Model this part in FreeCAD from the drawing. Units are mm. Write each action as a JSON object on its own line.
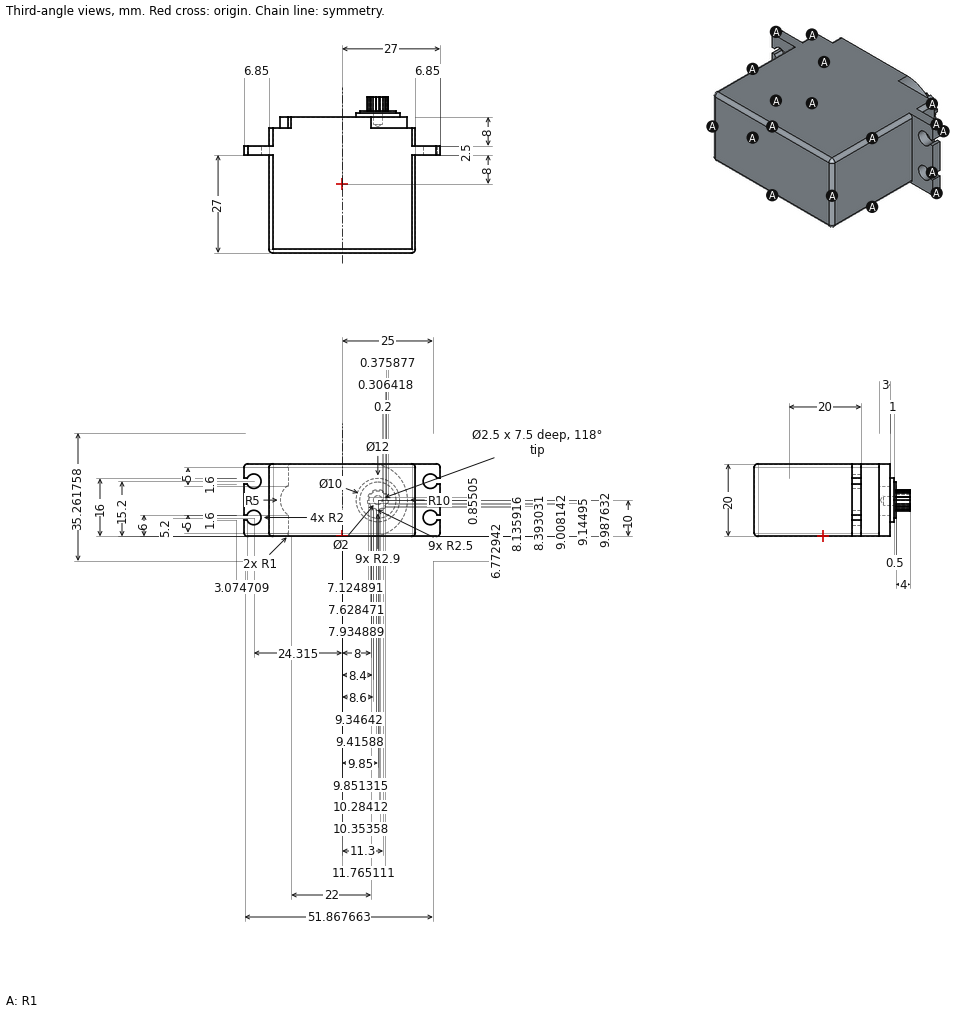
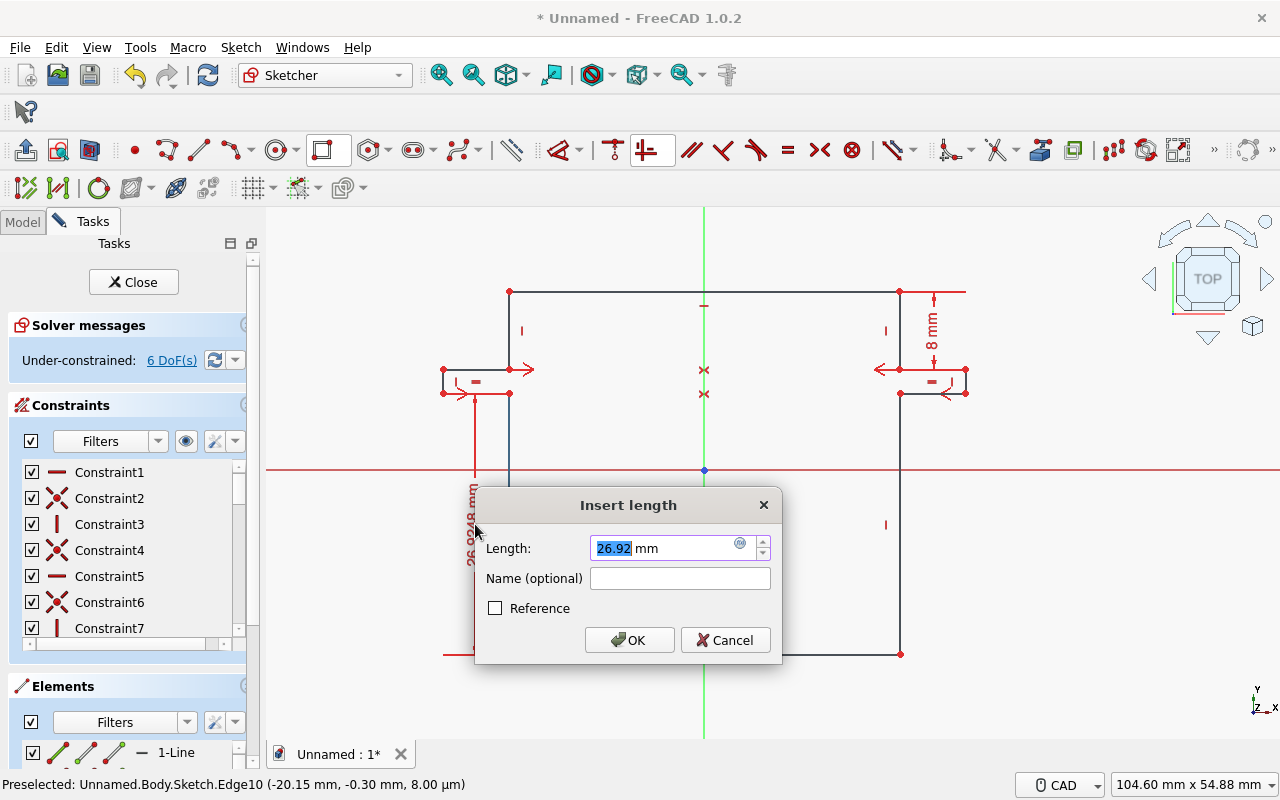
{"action": "type", "text": "27"}
{"action": "key", "text": "Return"}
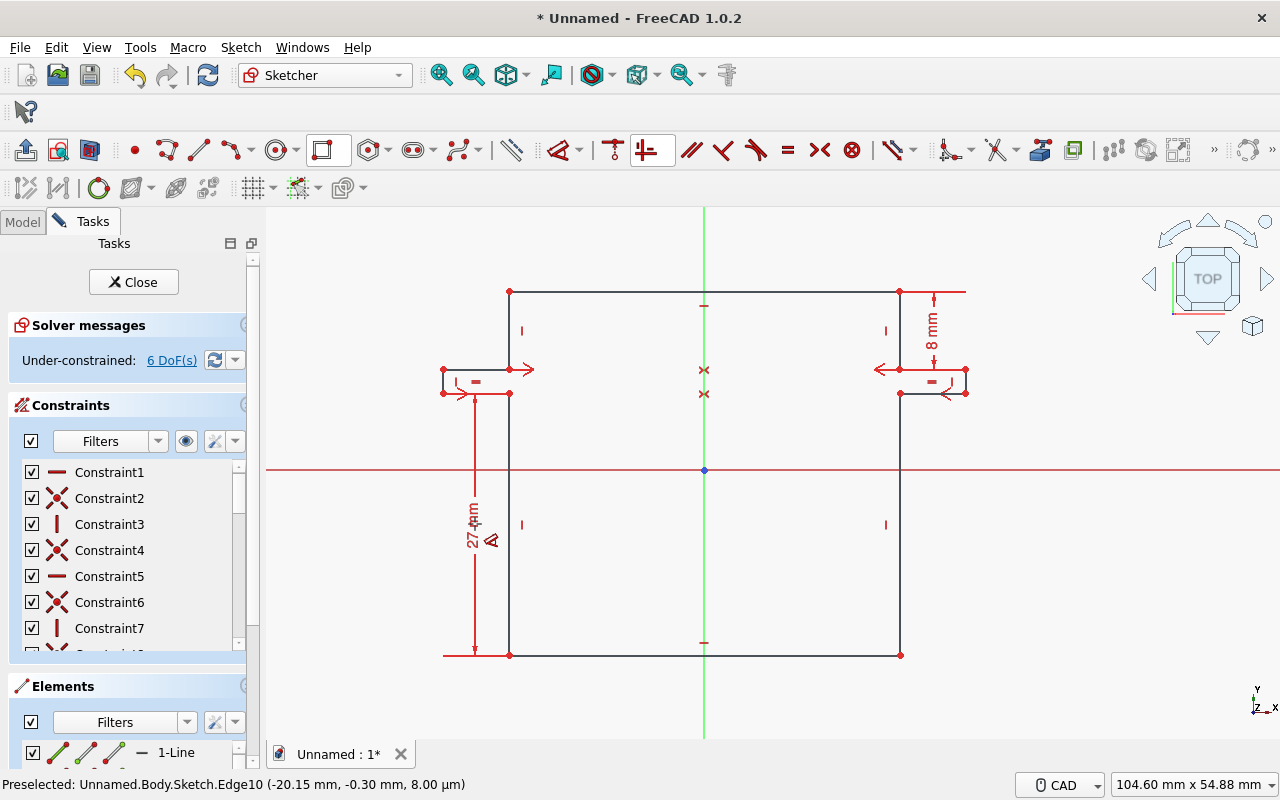
{"action": "left_click", "coordinate": [900, 394]}
{"action": "left_click", "coordinate": [934, 432]}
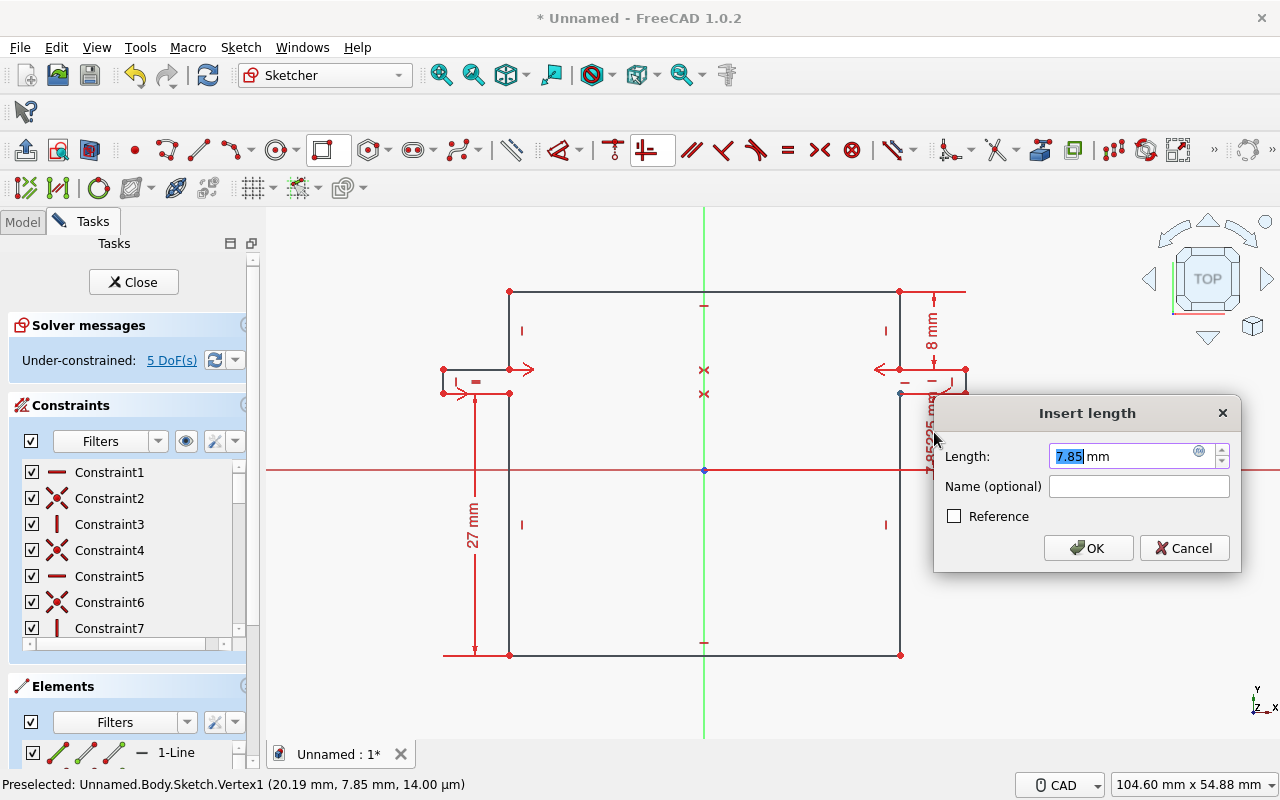
{"action": "type", "text": "8"}
{"action": "key", "text": "Return"}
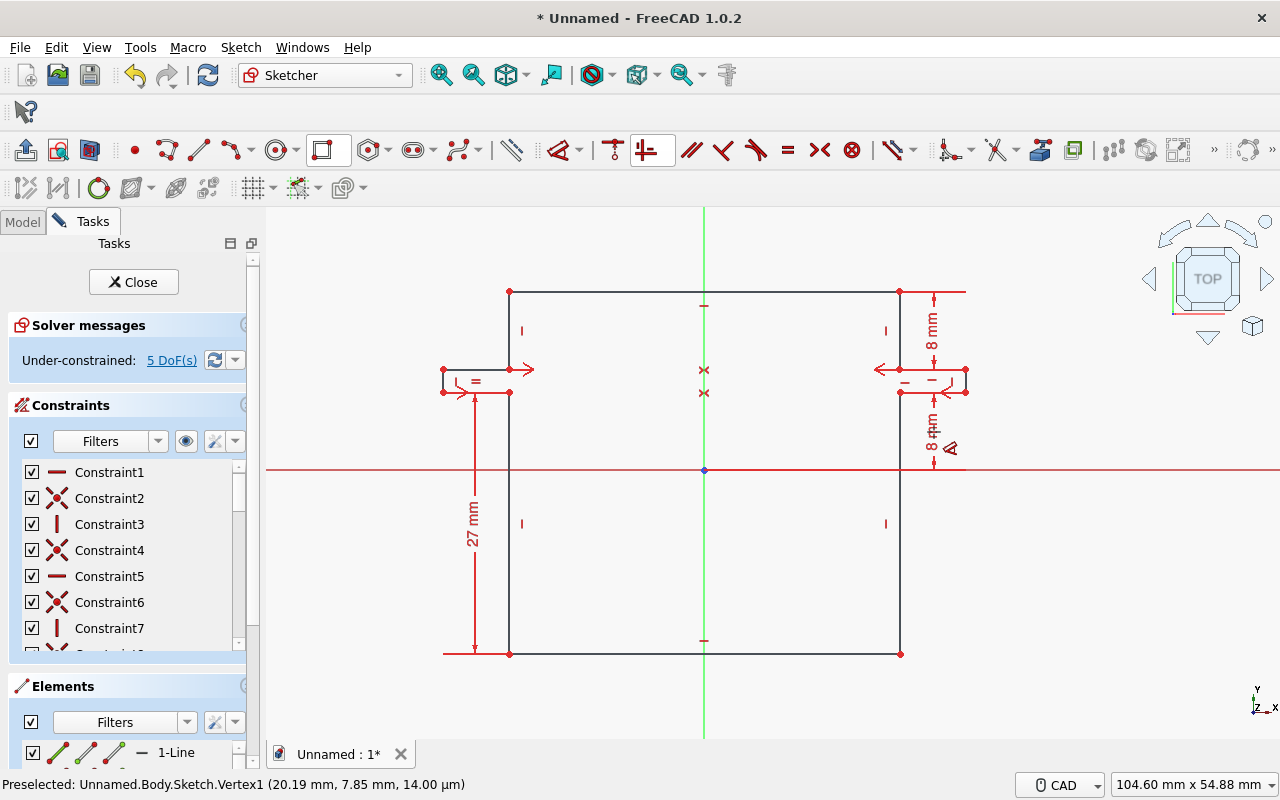
{"action": "scroll", "coordinate": [966, 383], "scroll_direction": "up", "scroll_amount": 3}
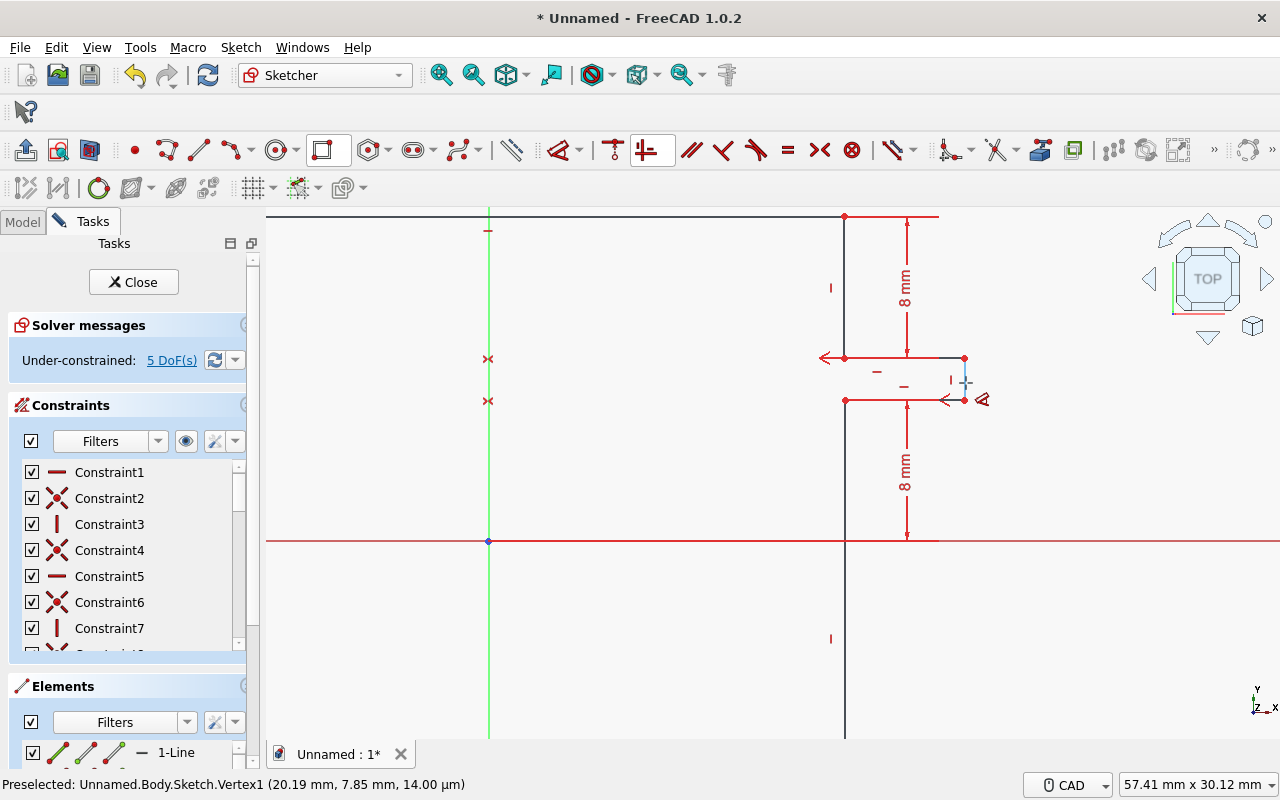
{"action": "left_click", "coordinate": [965, 383]}
{"action": "left_click", "coordinate": [999, 379]}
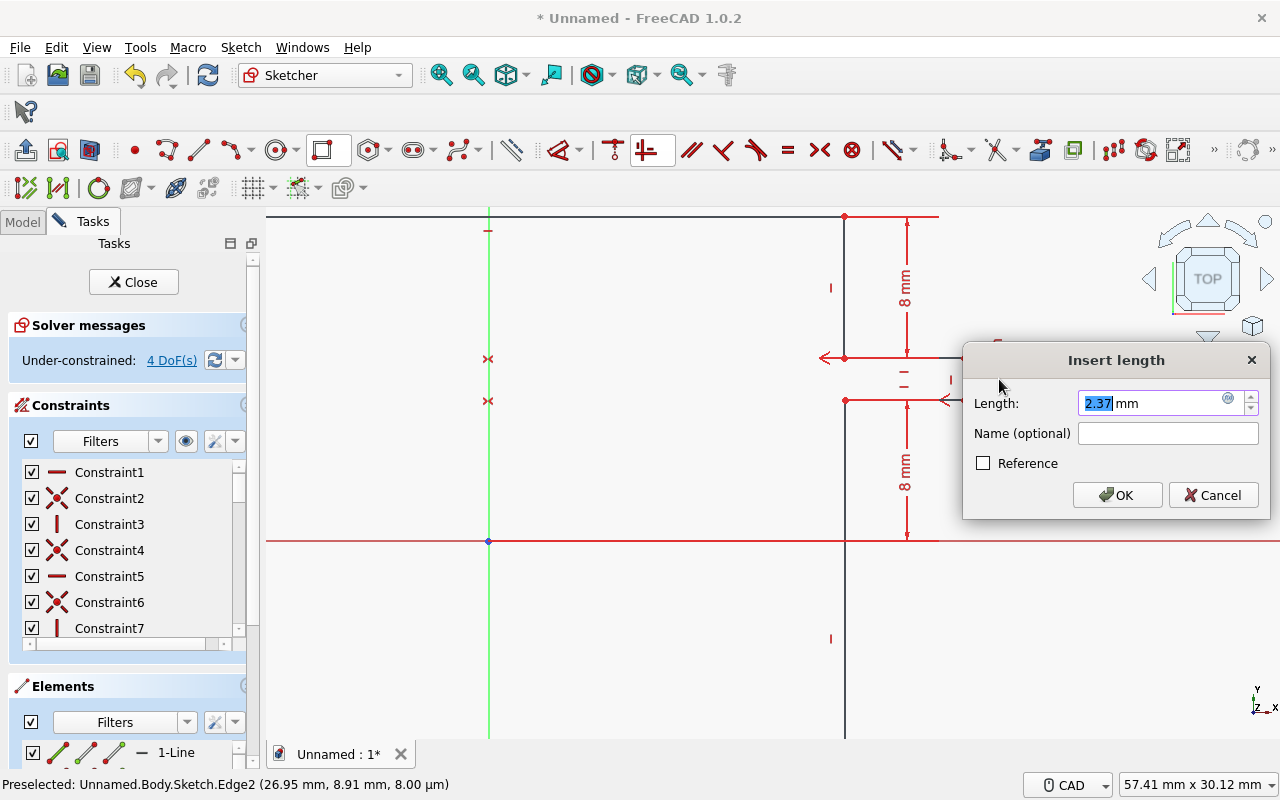
{"action": "type", "text": "2.5"}
{"action": "key", "text": "Return"}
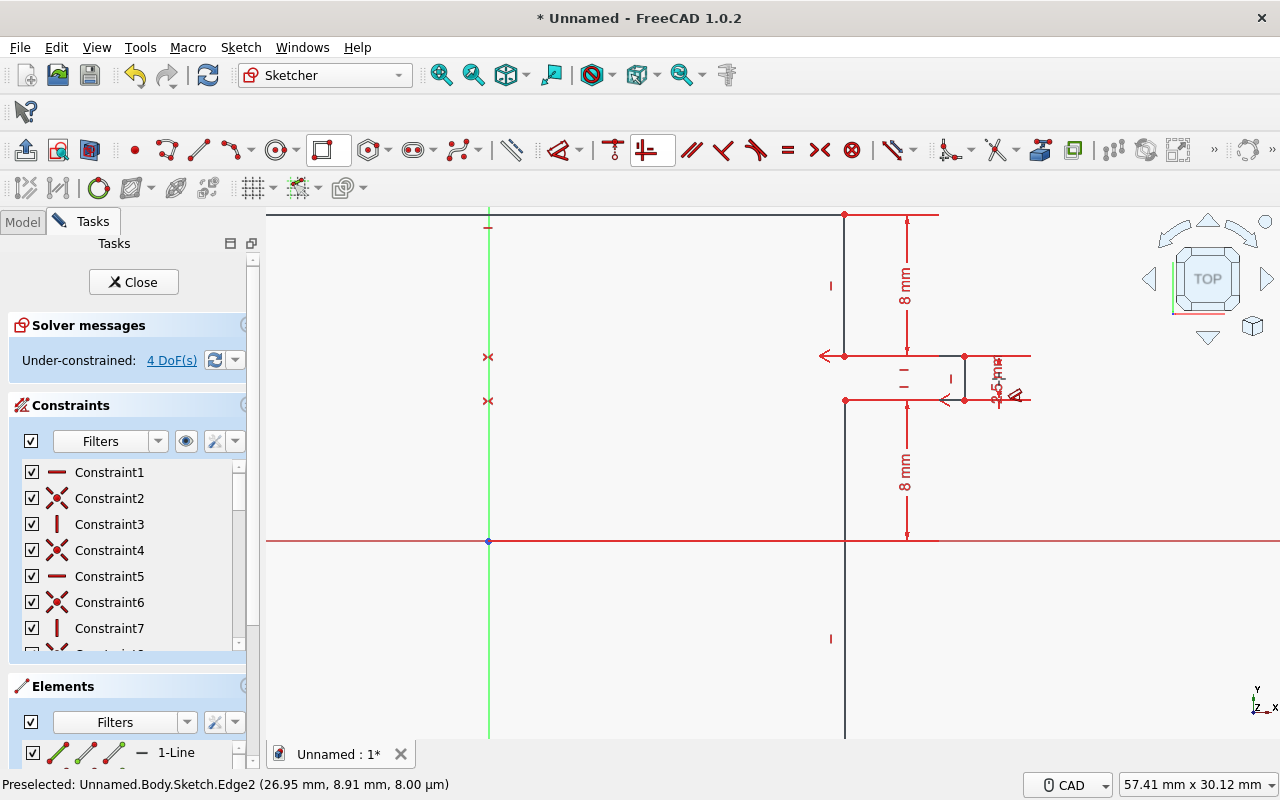
{"action": "left_click", "coordinate": [965, 400]}
{"action": "left_click", "coordinate": [727, 366]}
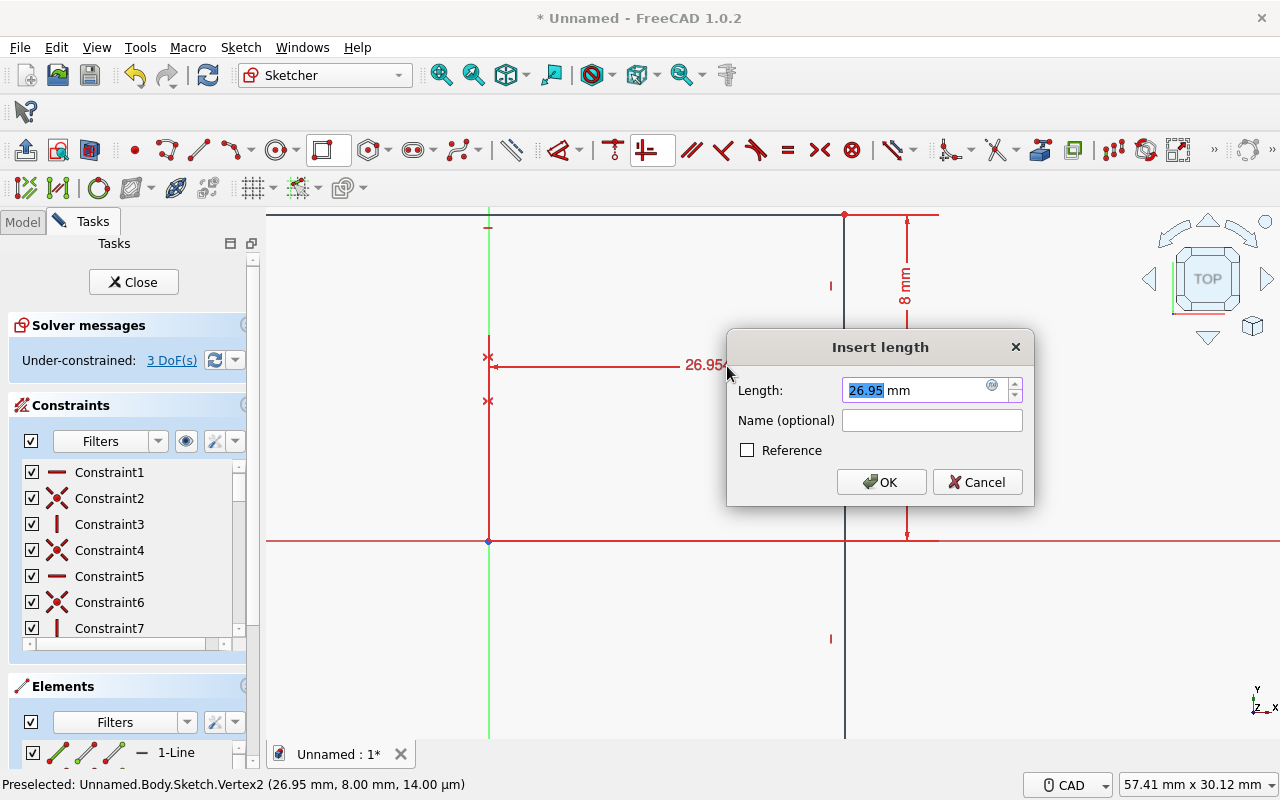
{"action": "type", "text": "27"}
{"action": "key", "text": "Return"}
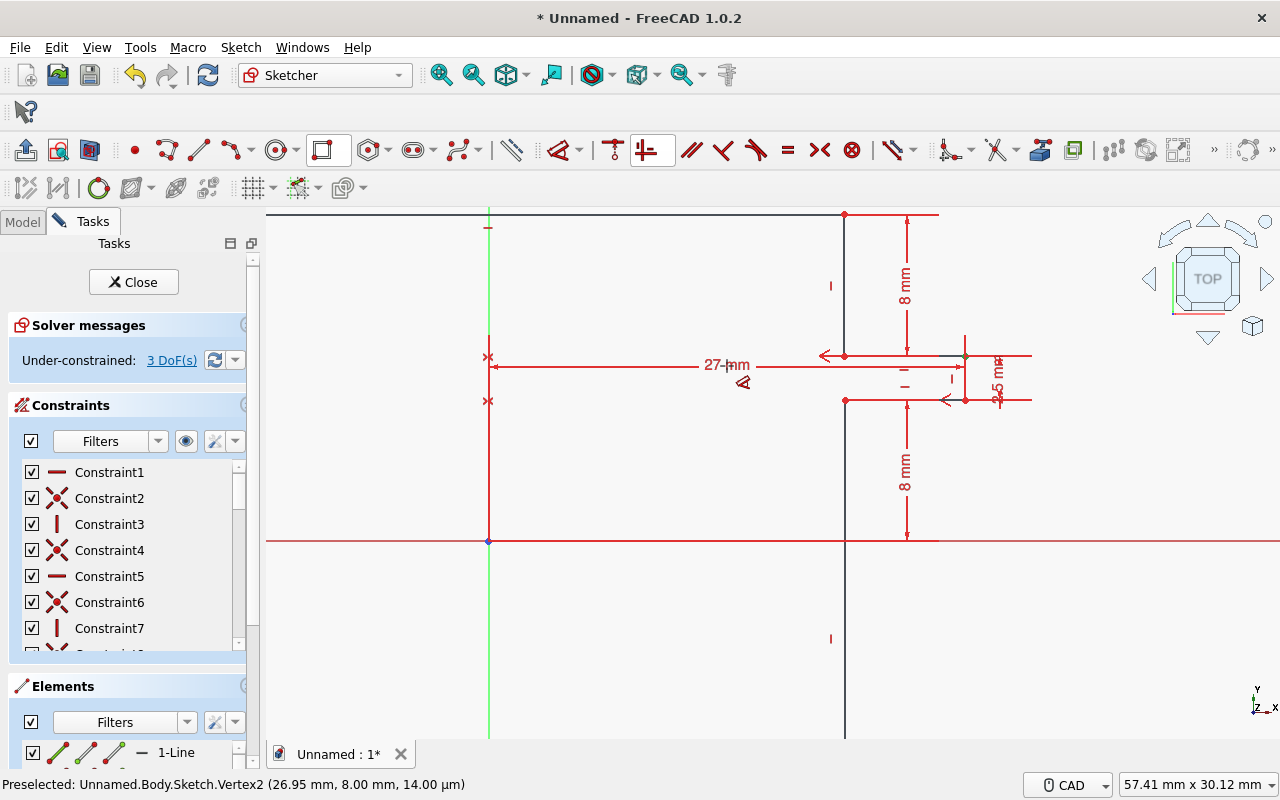
{"action": "left_click", "coordinate": [881, 400]}
{"action": "left_click", "coordinate": [905, 434]}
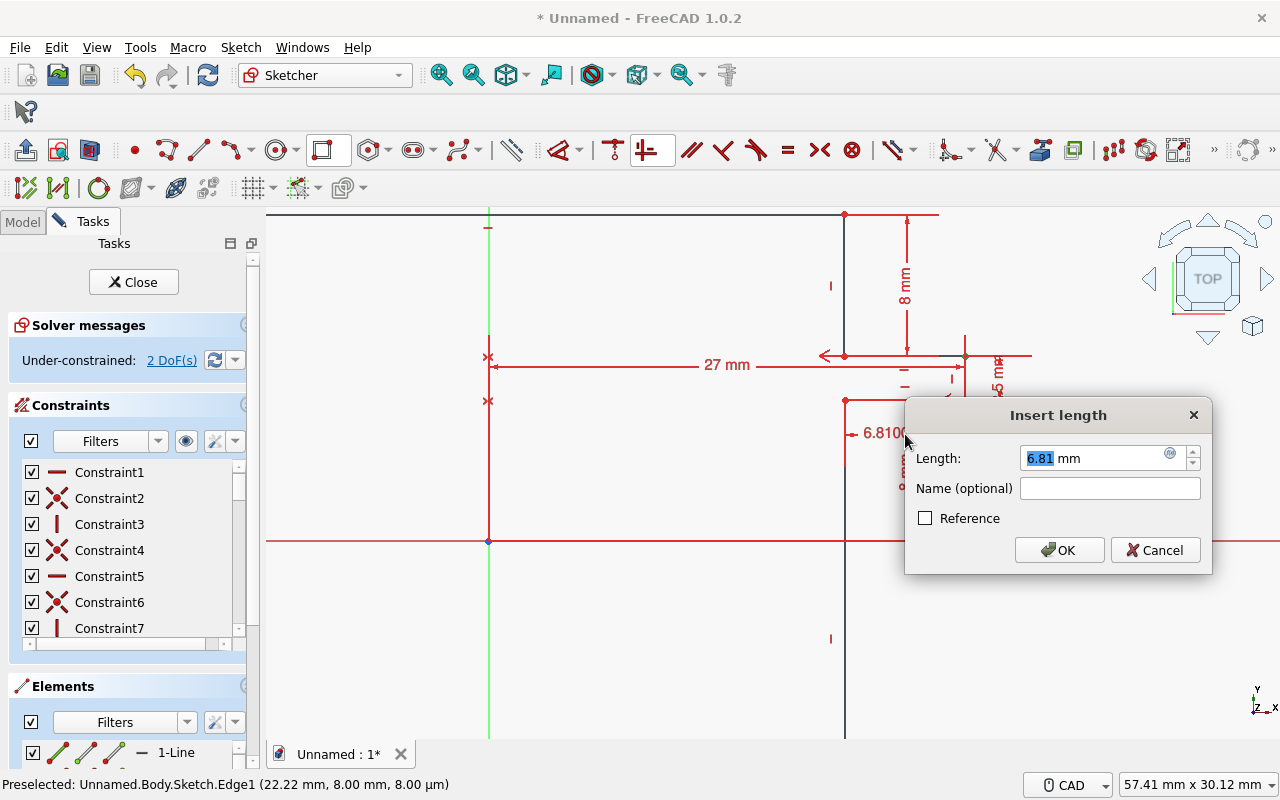
{"action": "type", "text": "6.85"}
{"action": "key", "text": "Return"}